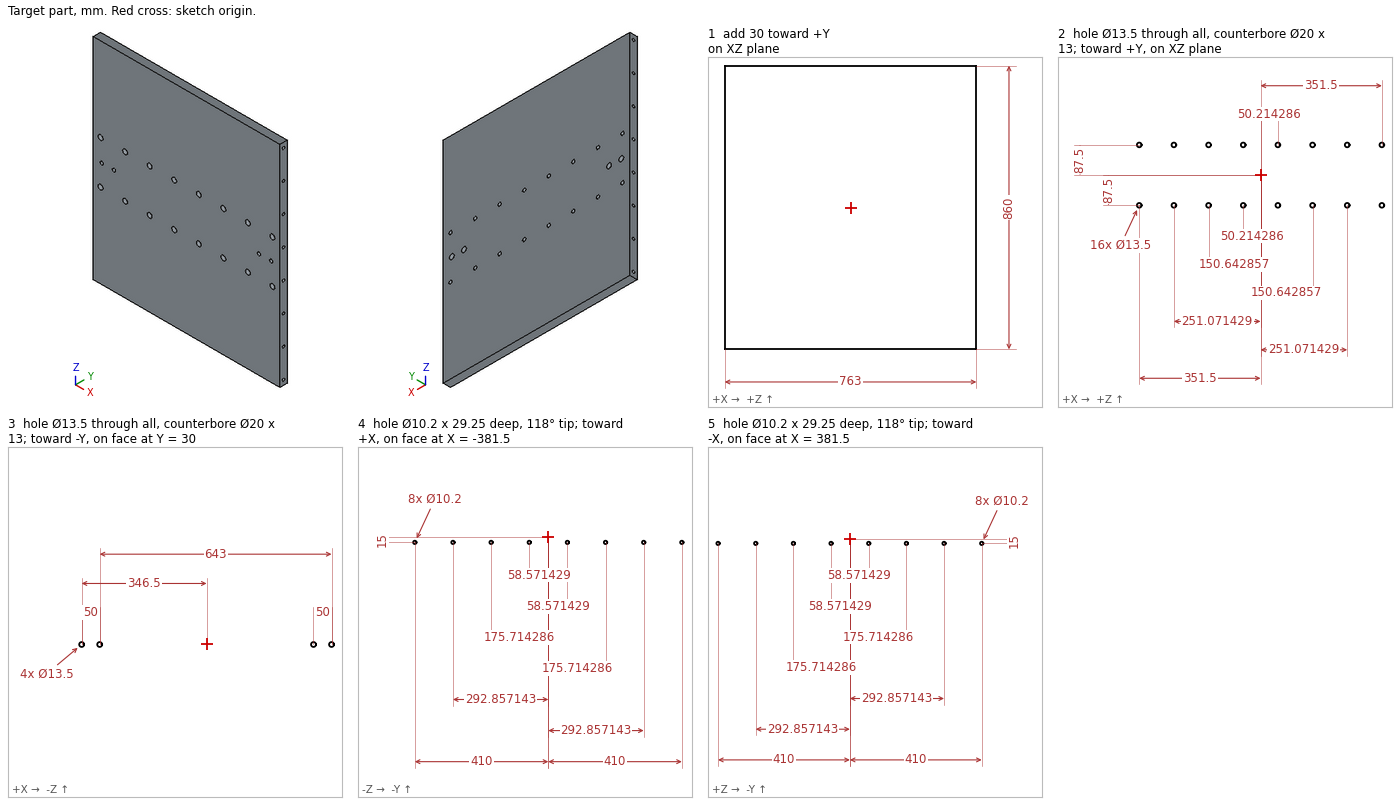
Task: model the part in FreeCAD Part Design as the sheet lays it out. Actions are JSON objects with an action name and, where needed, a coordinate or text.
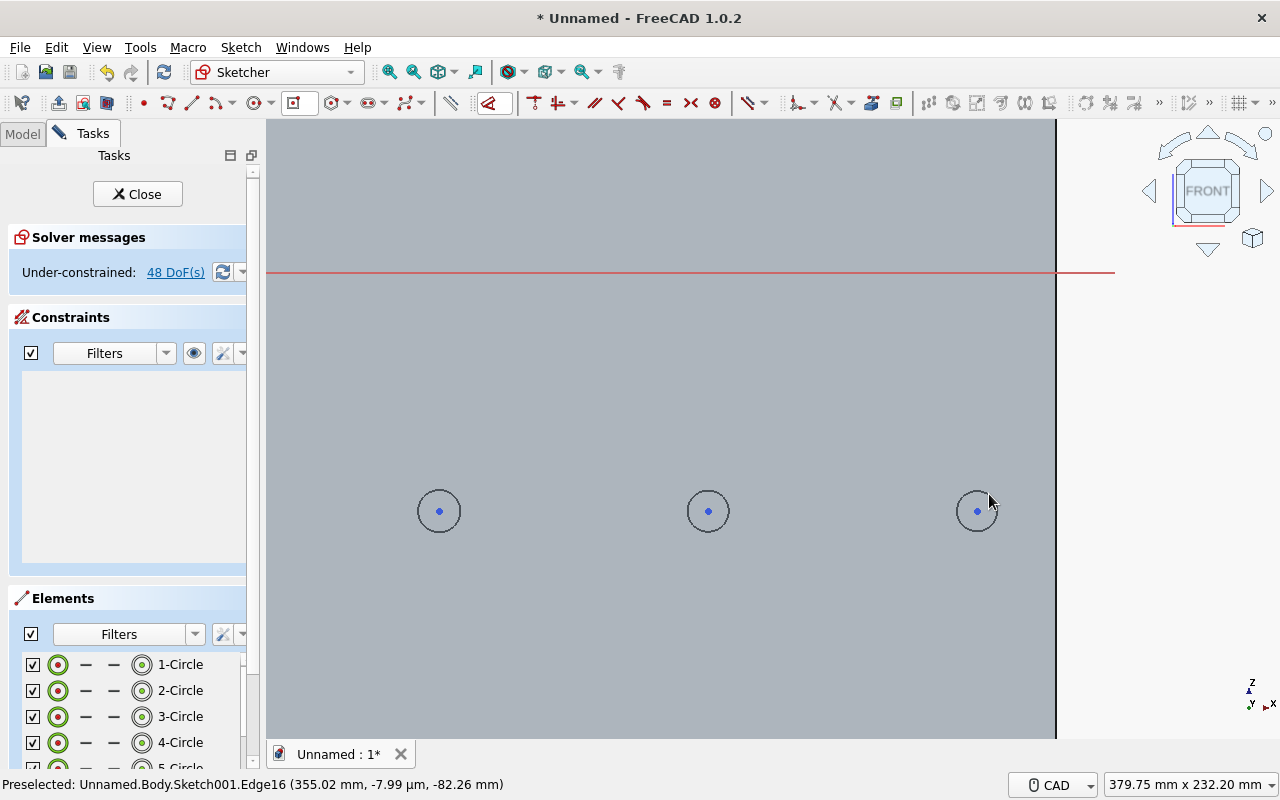
{"action": "scroll", "coordinate": [992, 496], "scroll_direction": "down", "scroll_amount": 6}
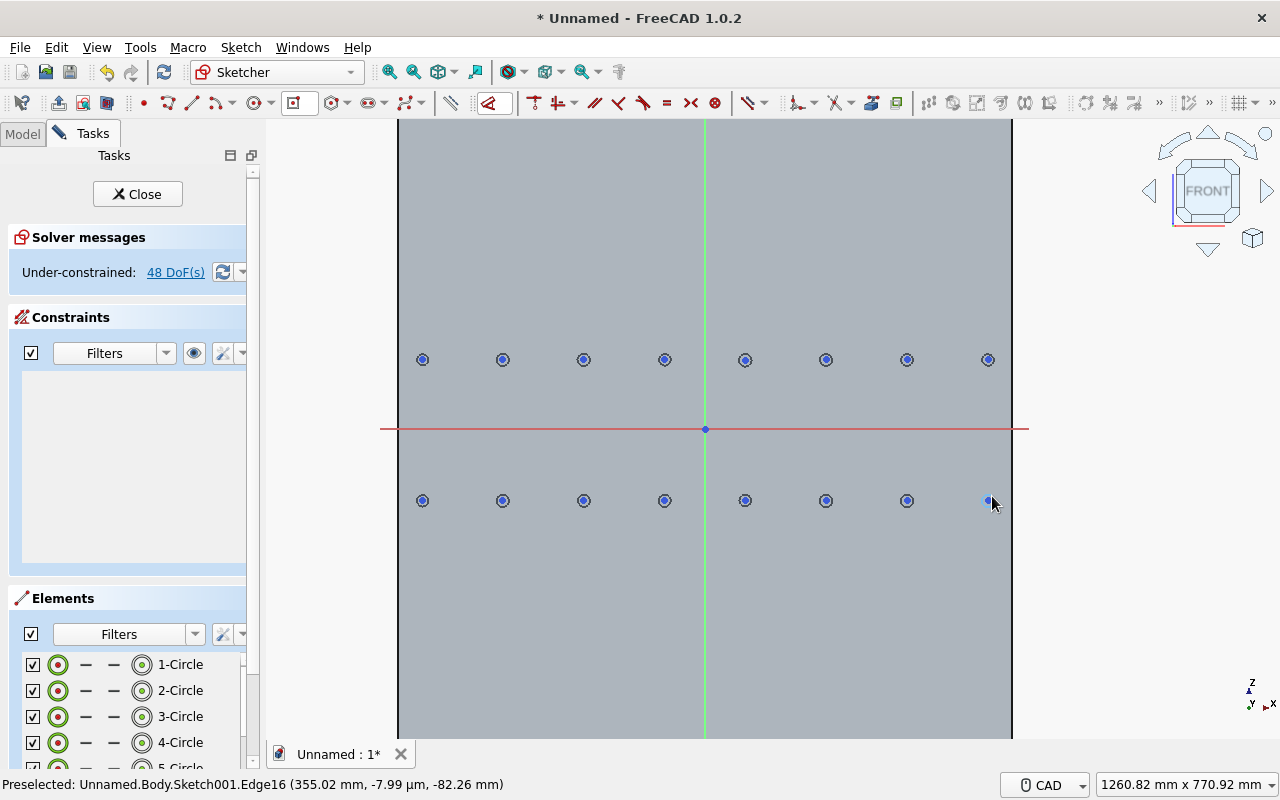
{"action": "scroll", "coordinate": [427, 497], "scroll_direction": "up", "scroll_amount": 5}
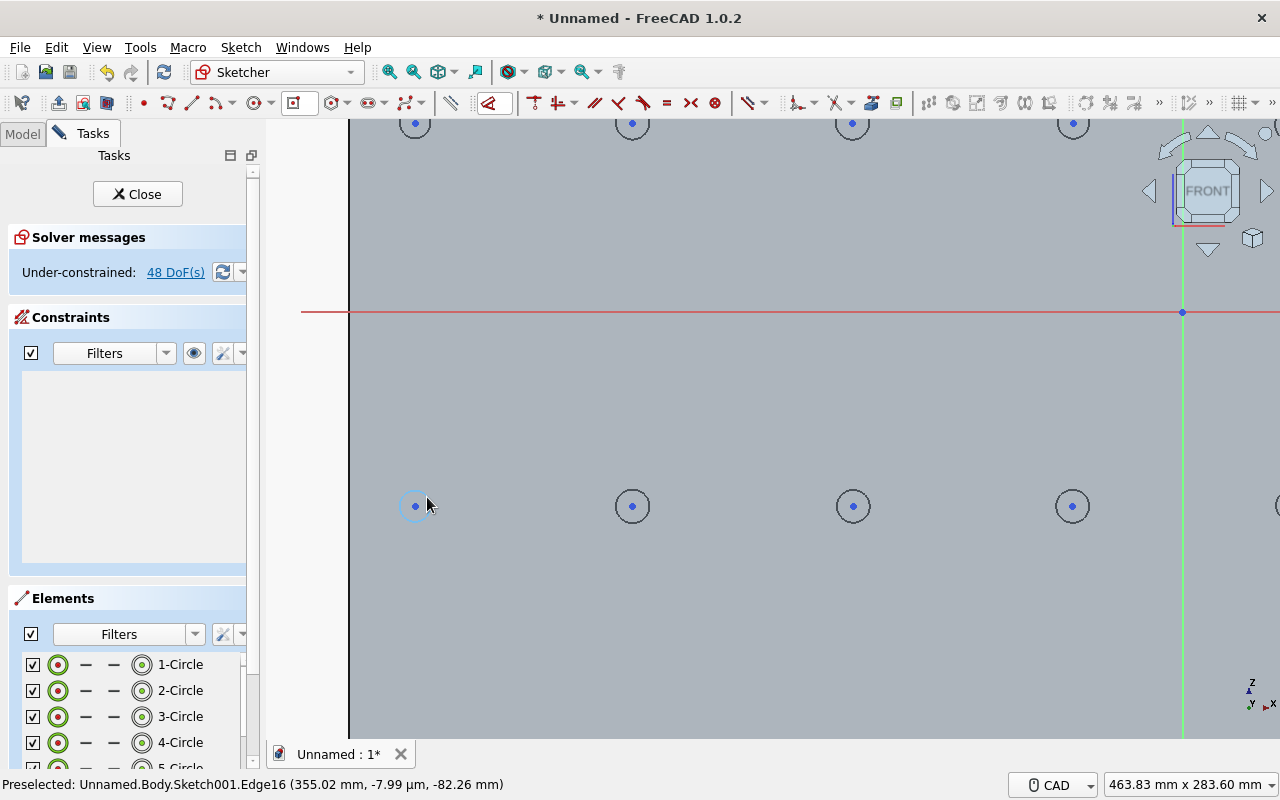
{"action": "left_click", "coordinate": [426, 495]}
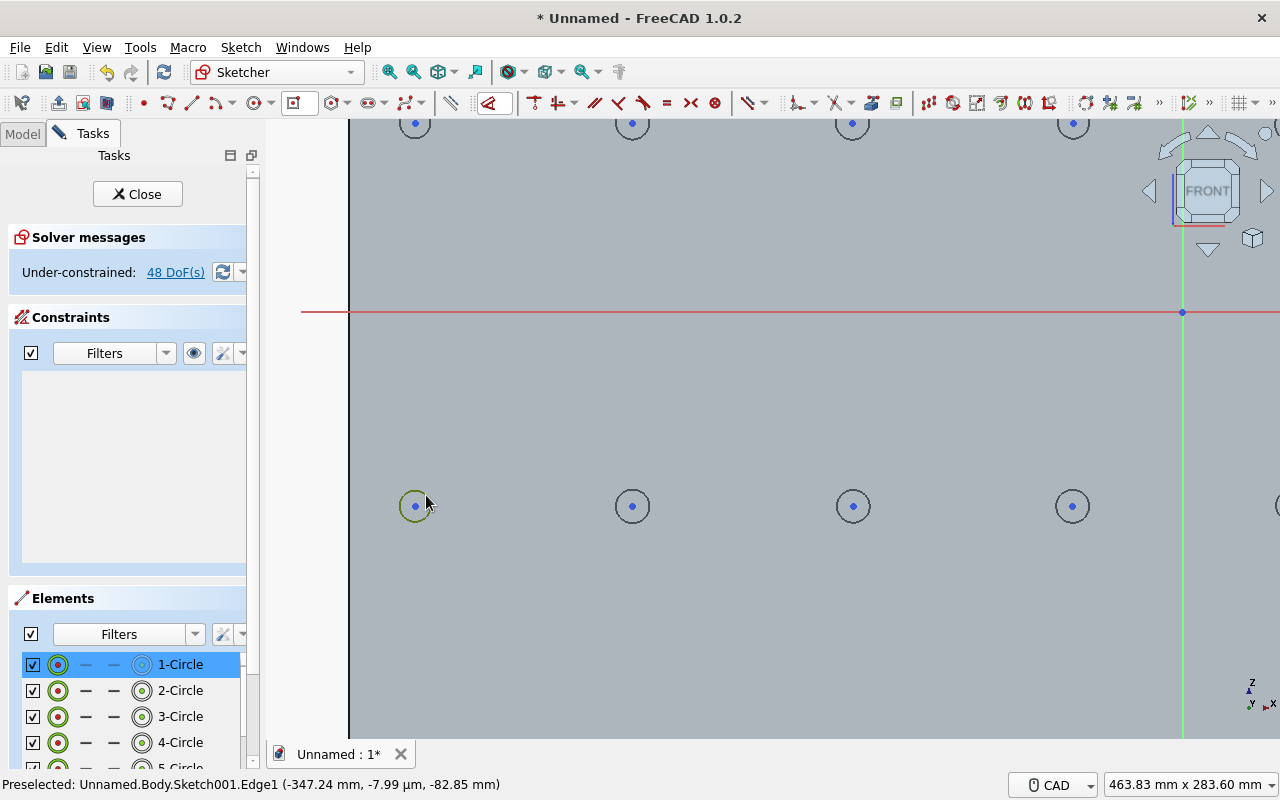
{"action": "scroll", "coordinate": [426, 497], "scroll_direction": "down", "scroll_amount": 5}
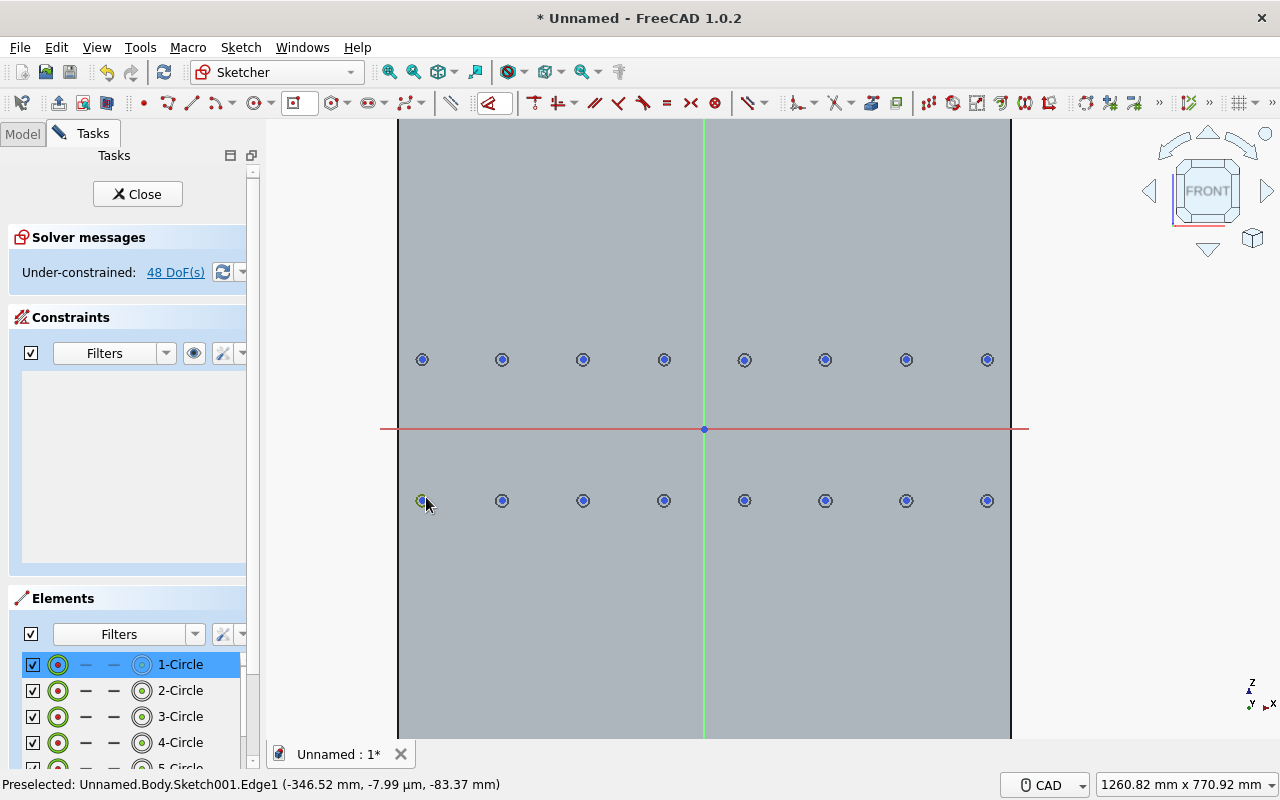
{"action": "scroll", "coordinate": [426, 356], "scroll_direction": "up", "scroll_amount": 5}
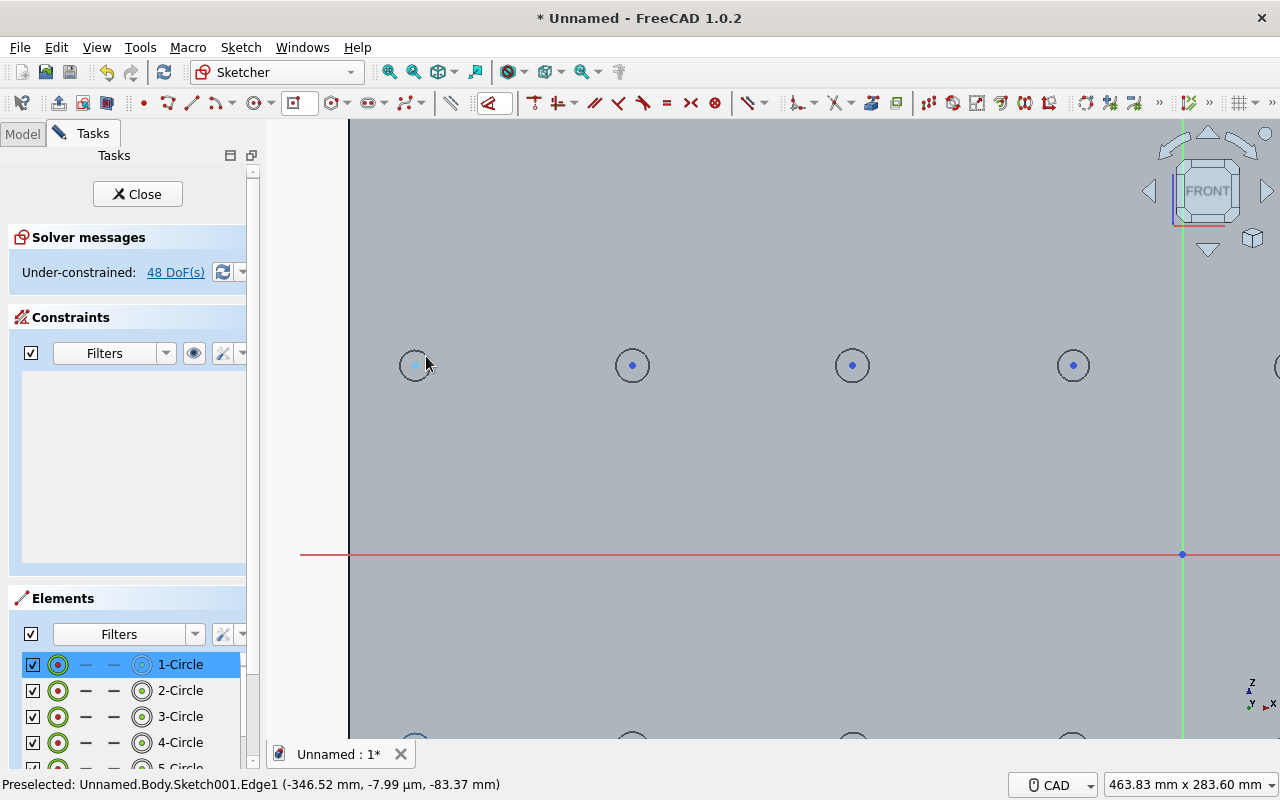
{"action": "left_click", "coordinate": [426, 355]}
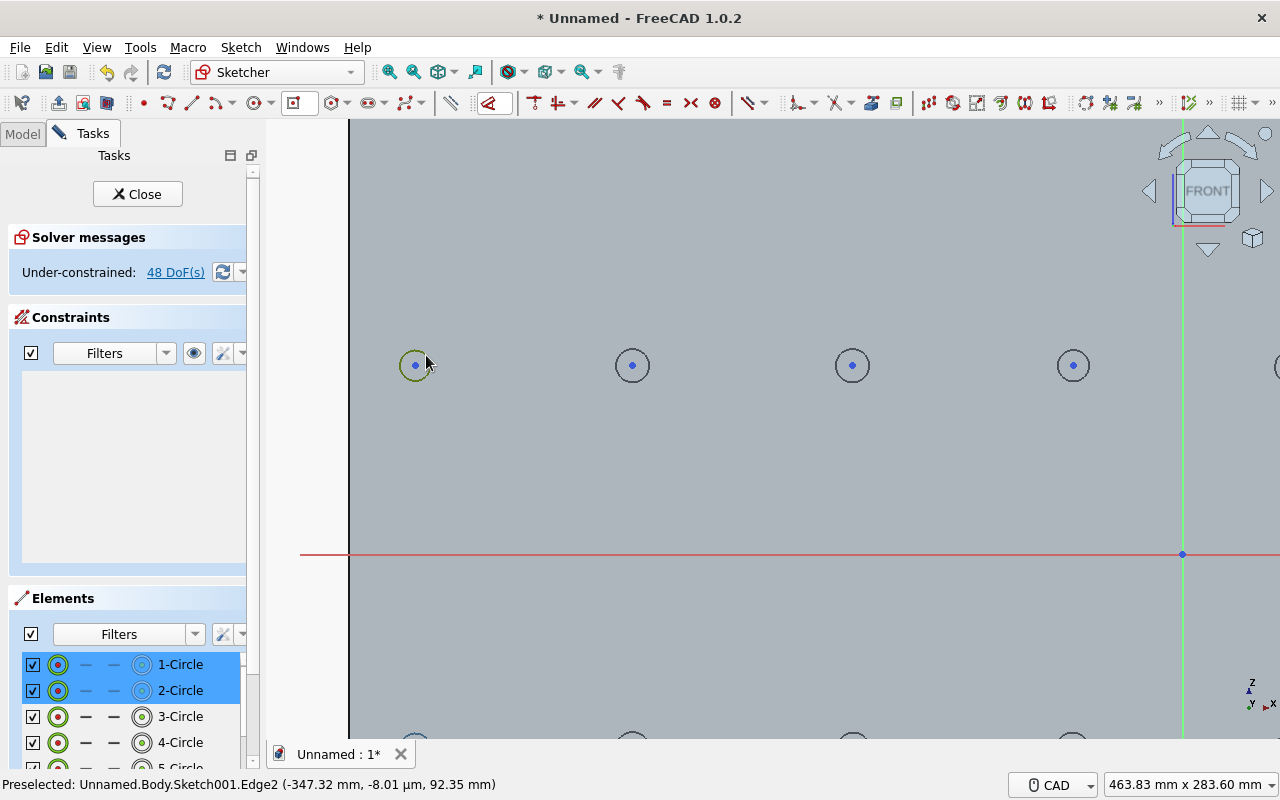
{"action": "scroll", "coordinate": [426, 356], "scroll_direction": "down", "scroll_amount": 5}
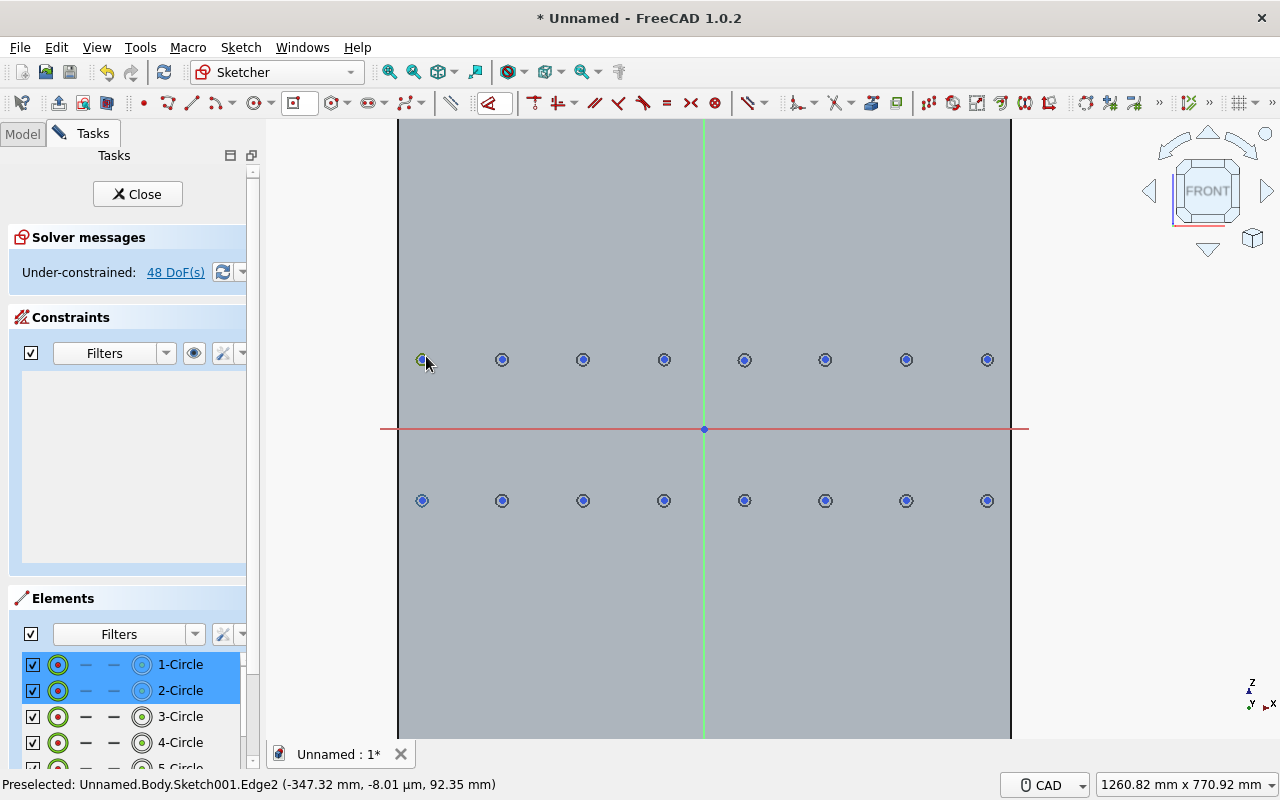
{"action": "scroll", "coordinate": [506, 496], "scroll_direction": "up", "scroll_amount": 5}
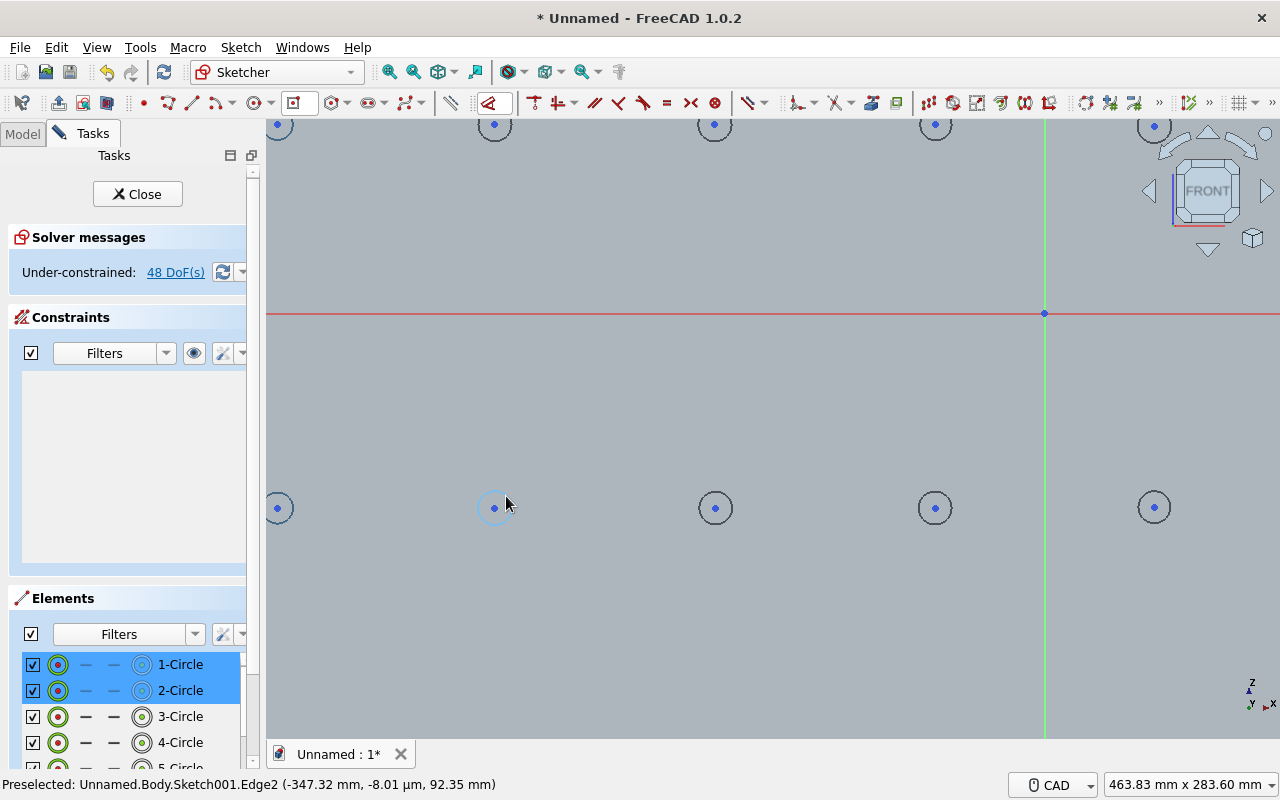
{"action": "left_click", "coordinate": [507, 496]}